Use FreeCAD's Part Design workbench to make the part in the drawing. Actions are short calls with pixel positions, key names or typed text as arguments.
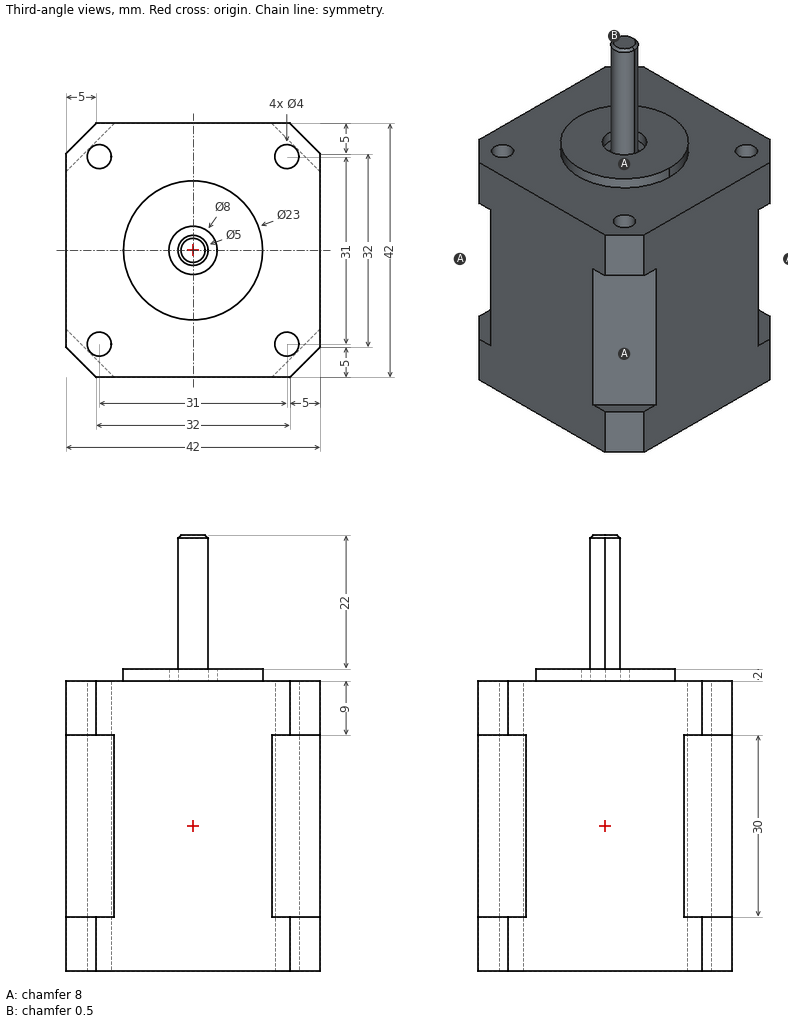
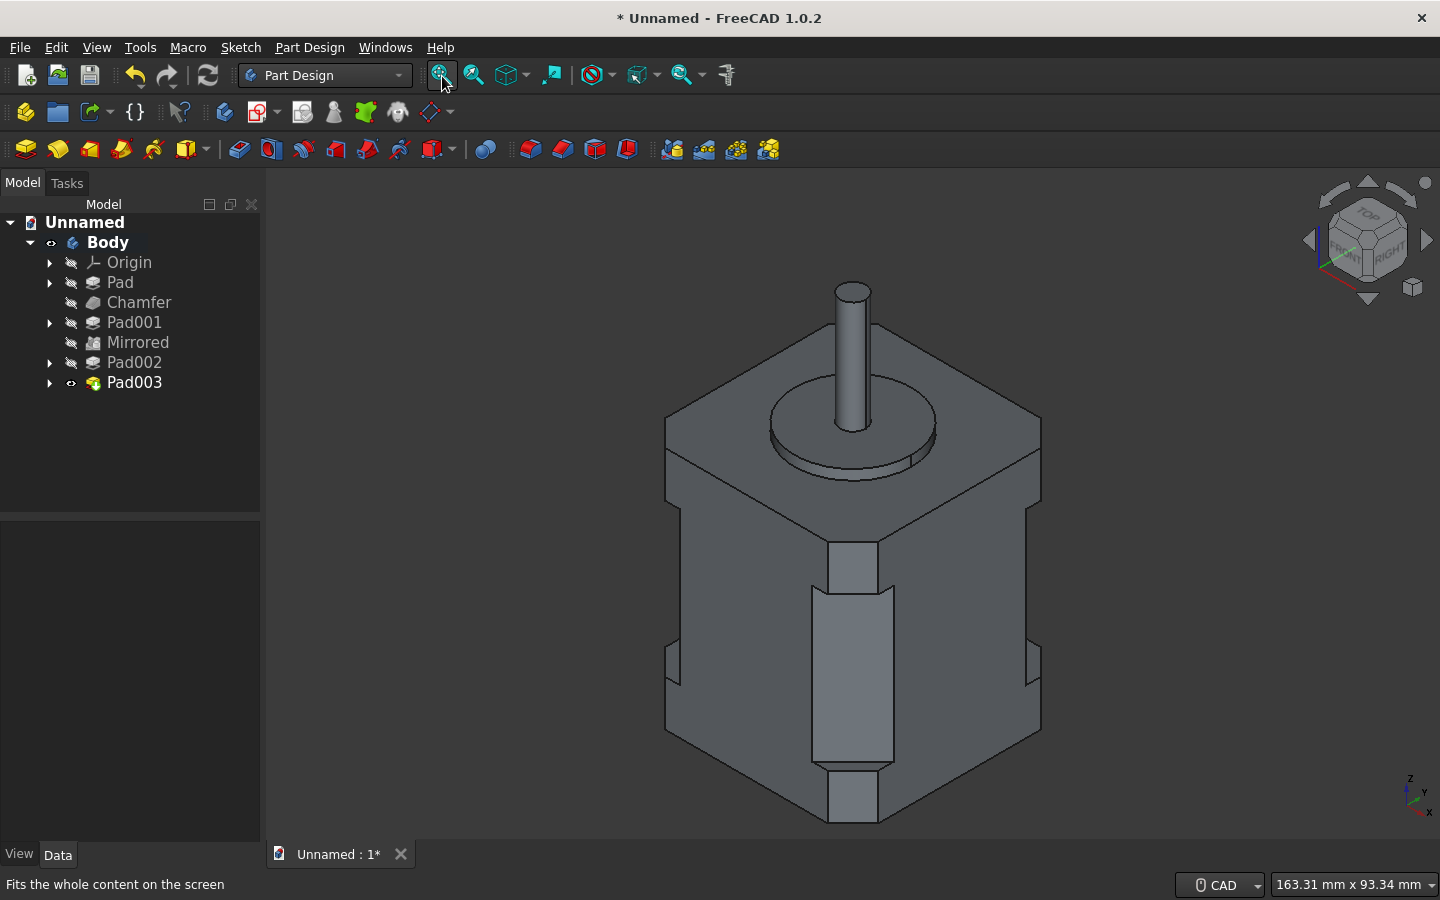
click(975, 432)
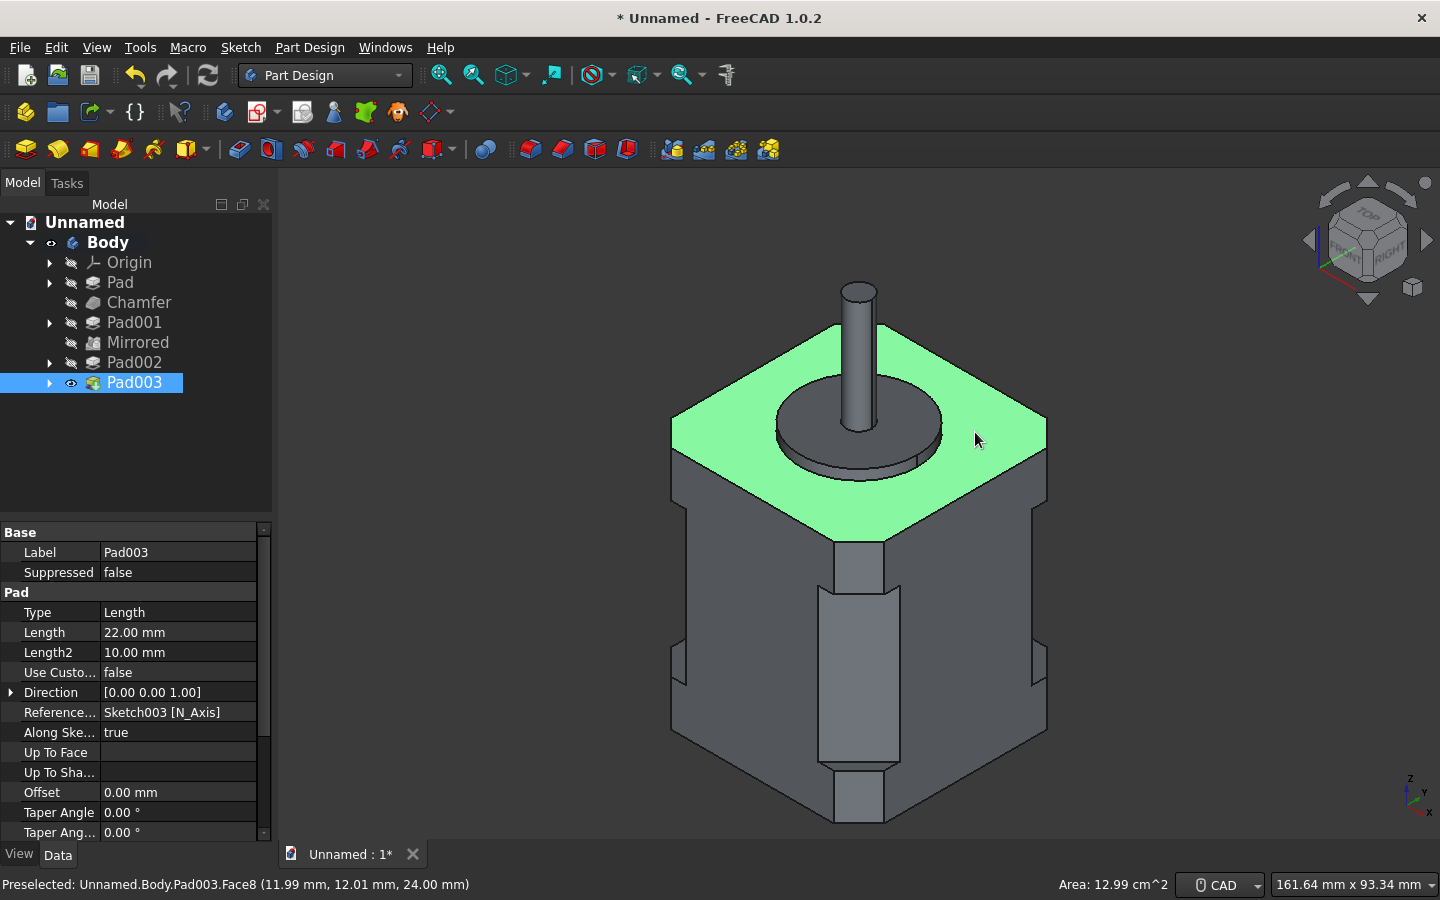
click(258, 112)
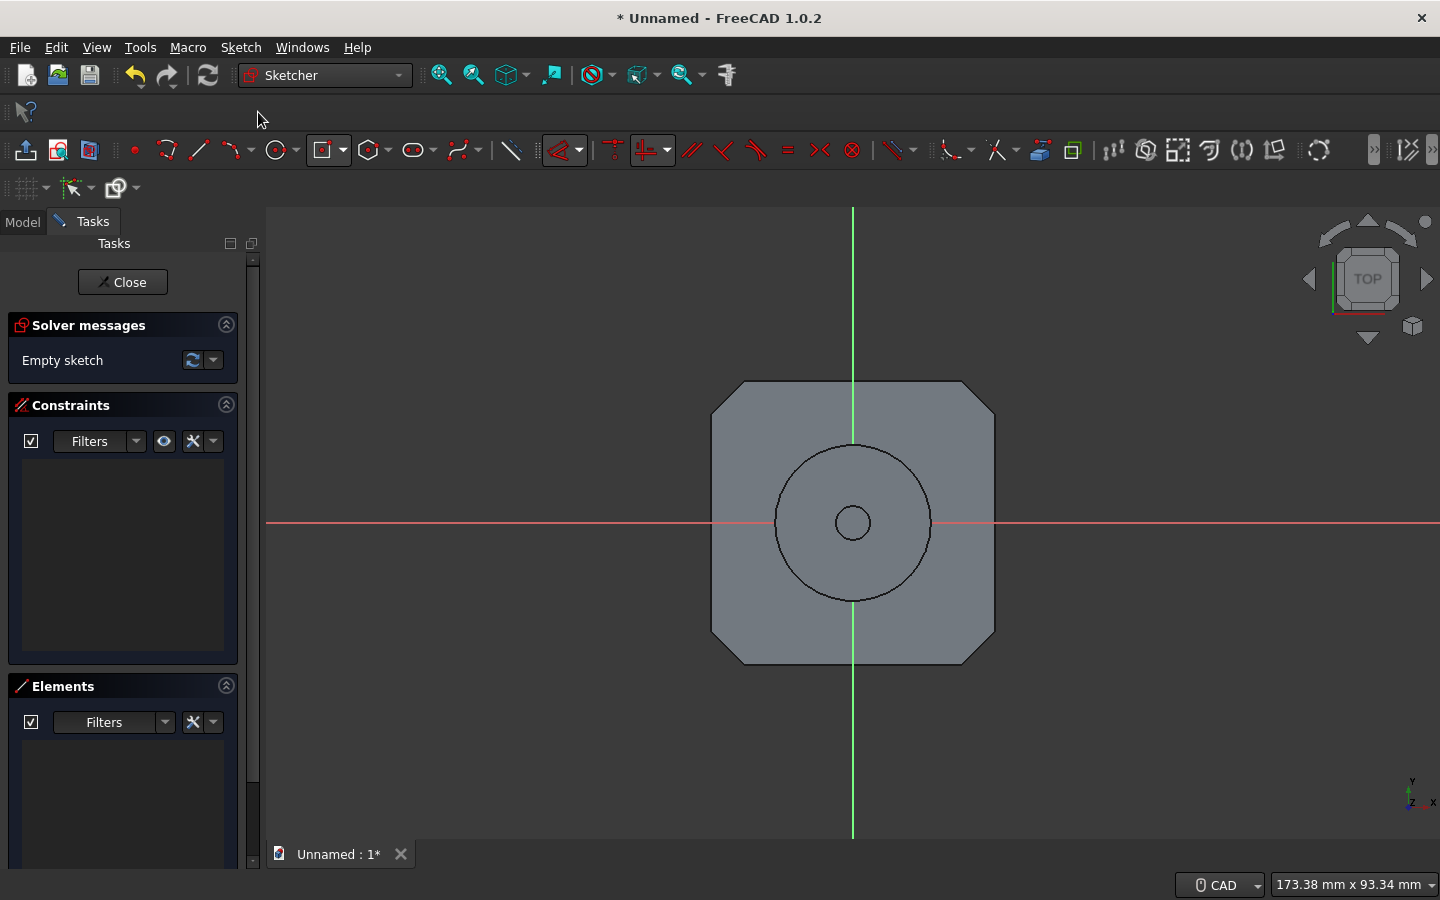
click(90, 150)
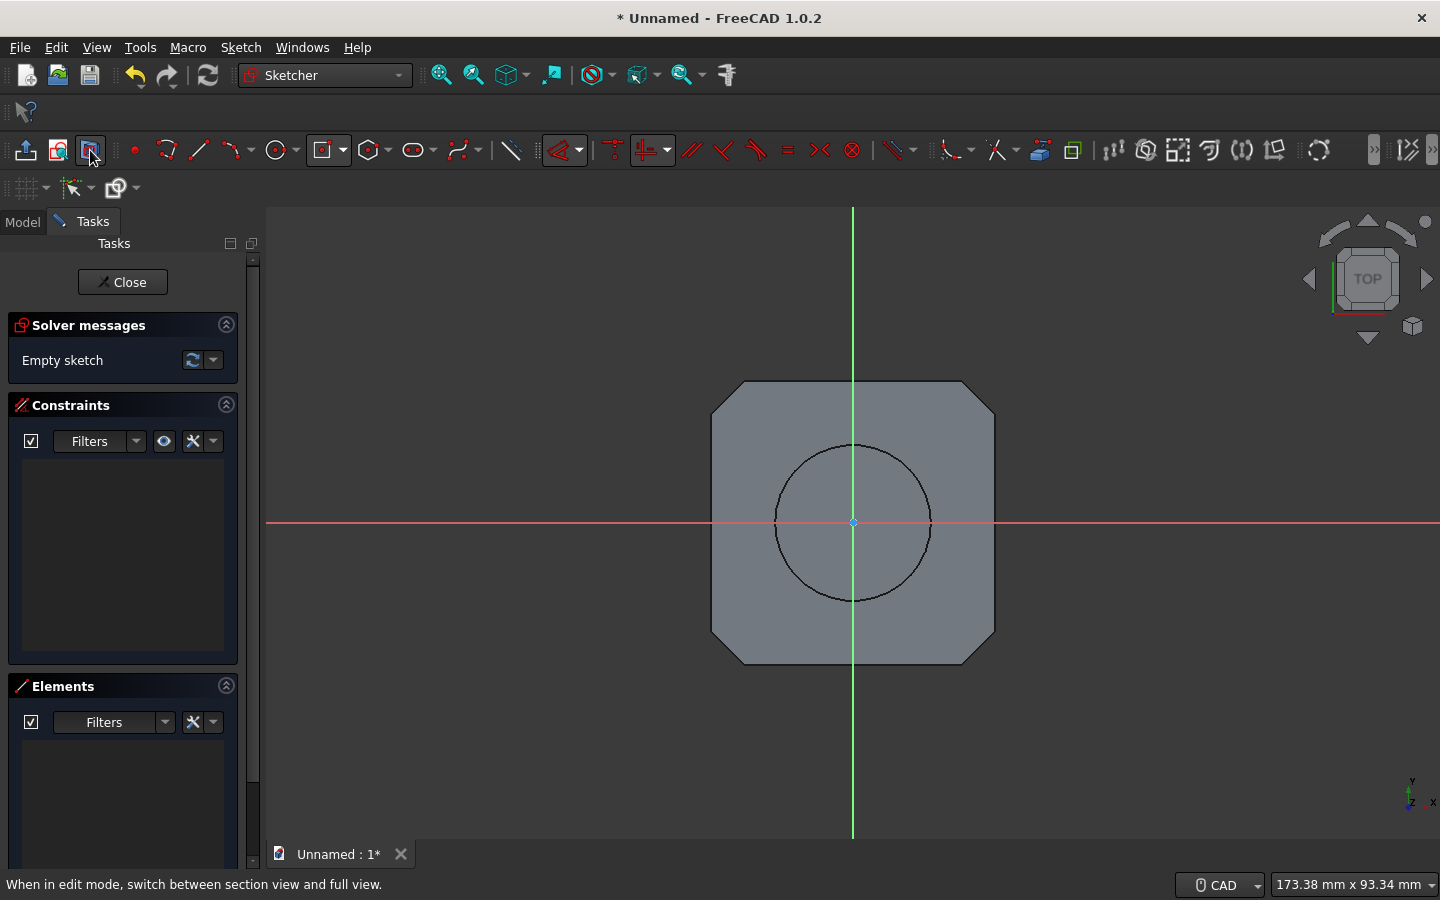
scroll(864, 523, up, 10)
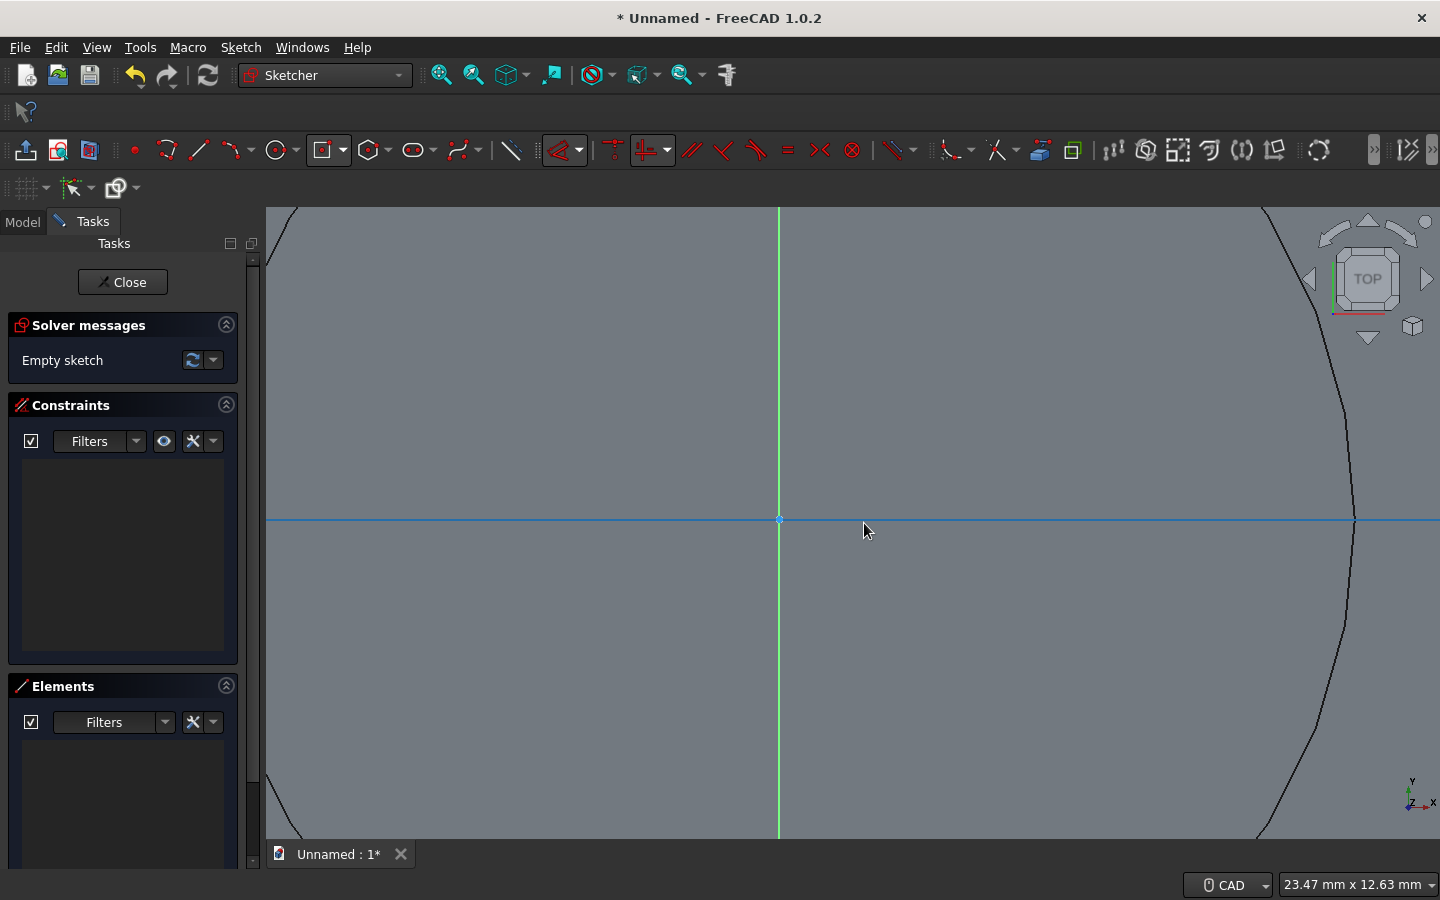
click(276, 150)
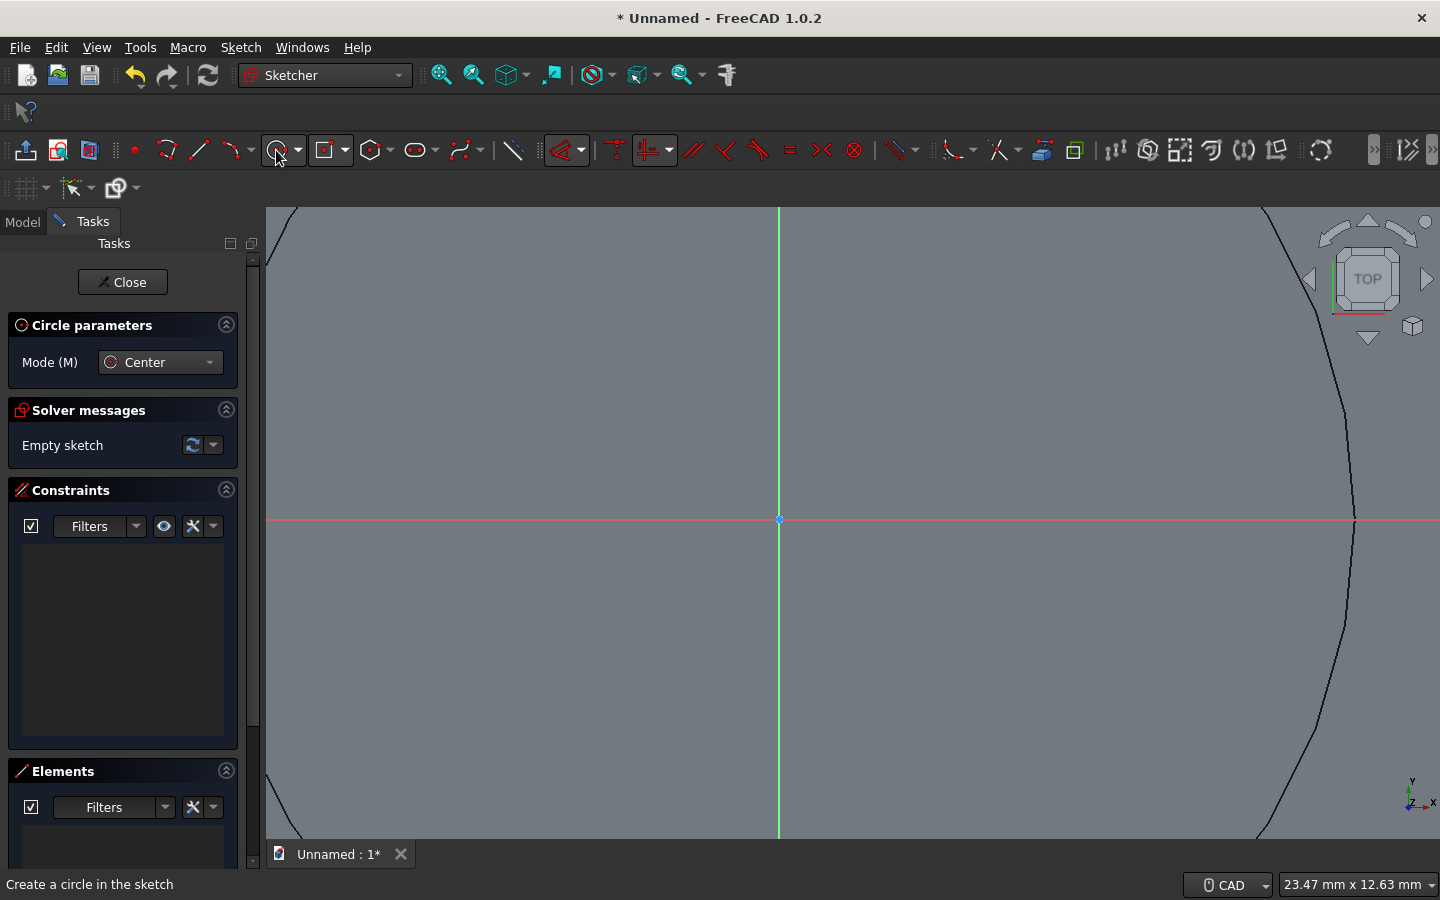
click(779, 520)
move(921, 378)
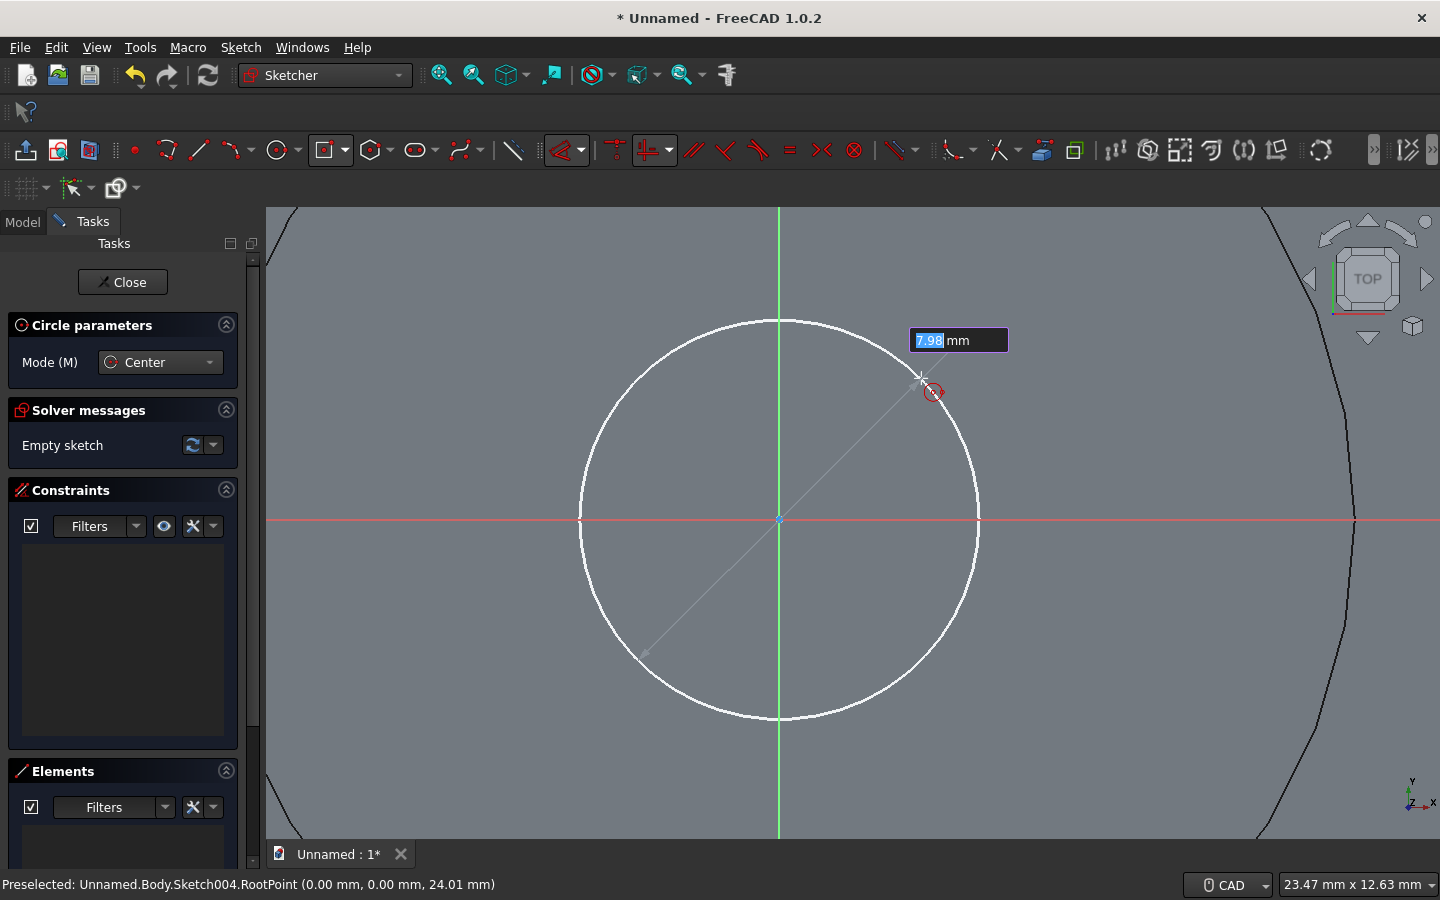
text(8)
key(Return)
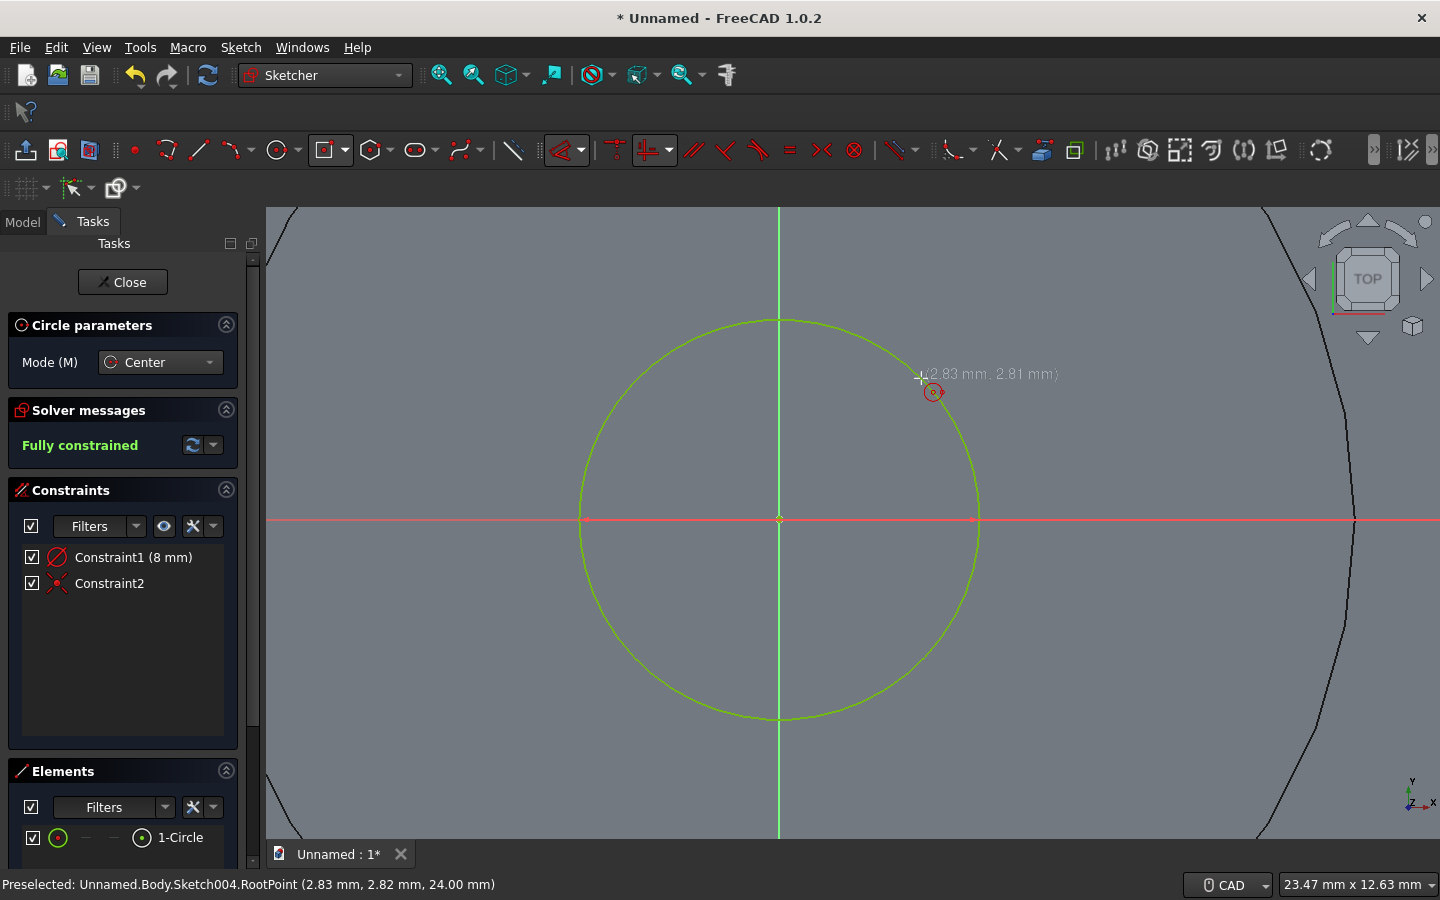
click(779, 520)
move(868, 431)